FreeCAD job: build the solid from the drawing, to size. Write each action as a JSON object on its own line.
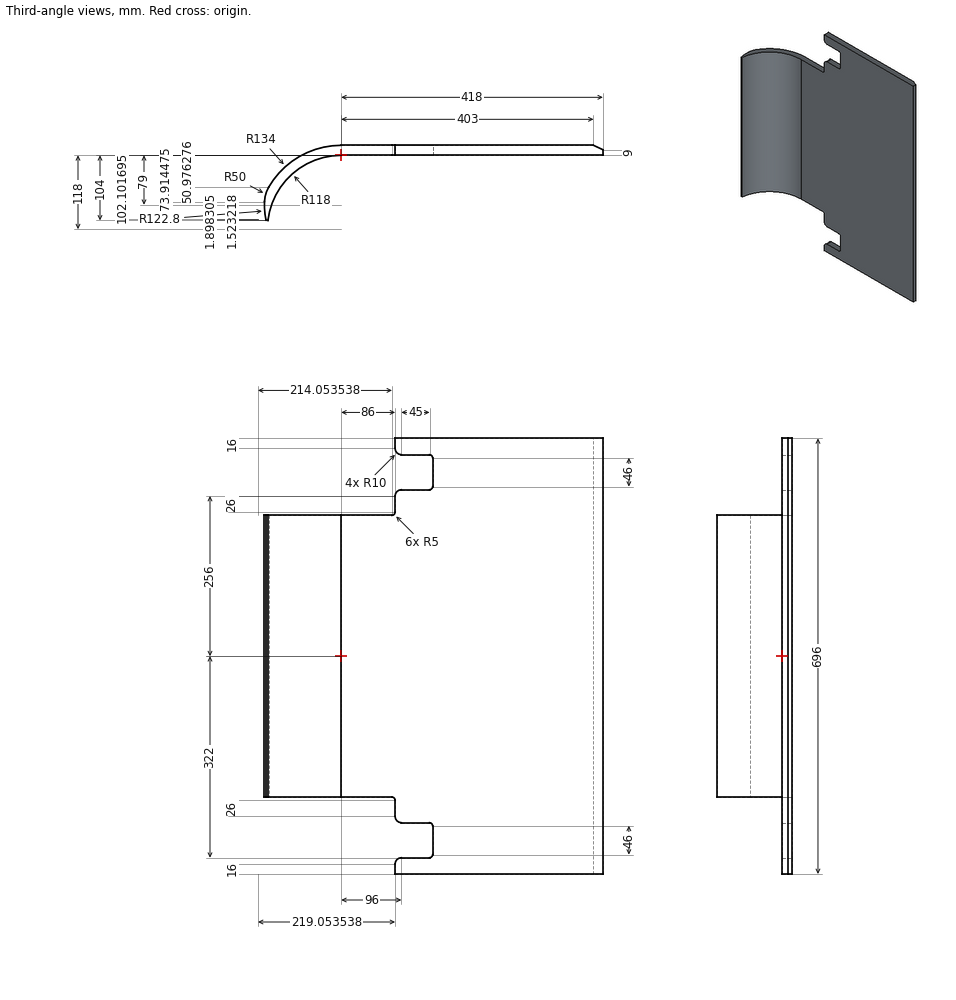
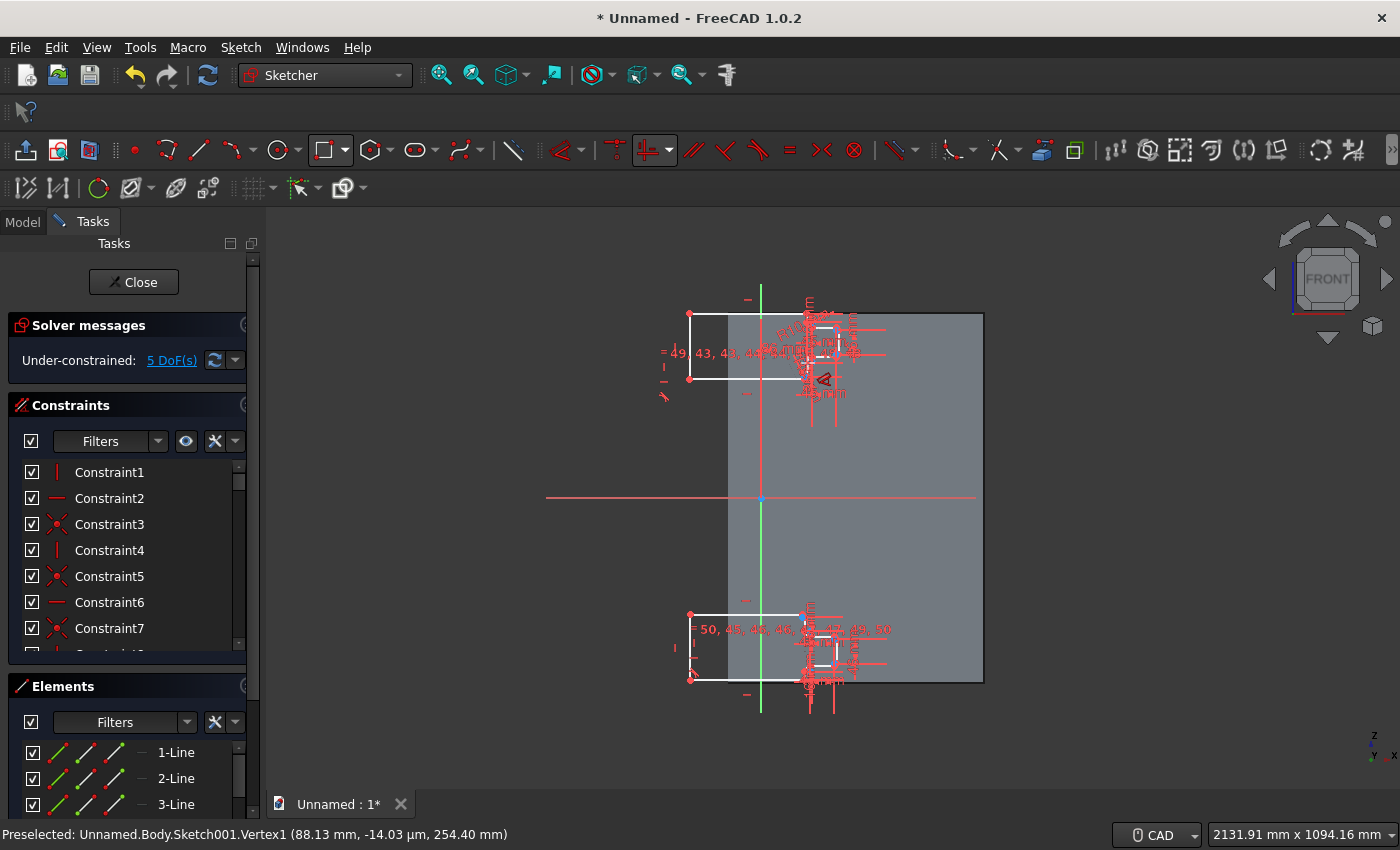
{"action": "scroll", "coordinate": [810, 666], "scroll_direction": "up", "scroll_amount": 5}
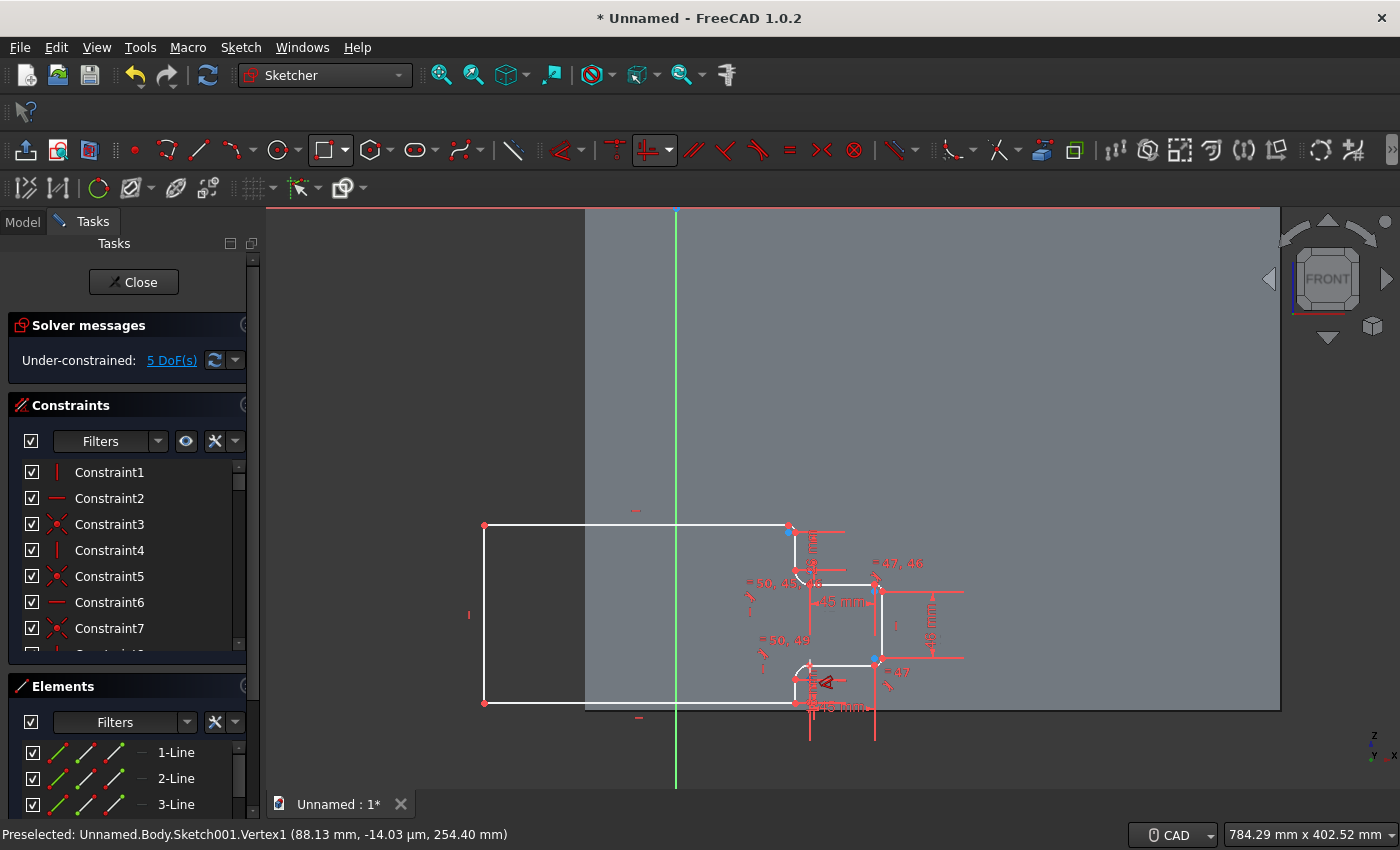
{"action": "left_click", "coordinate": [810, 666]}
{"action": "left_click", "coordinate": [712, 724]}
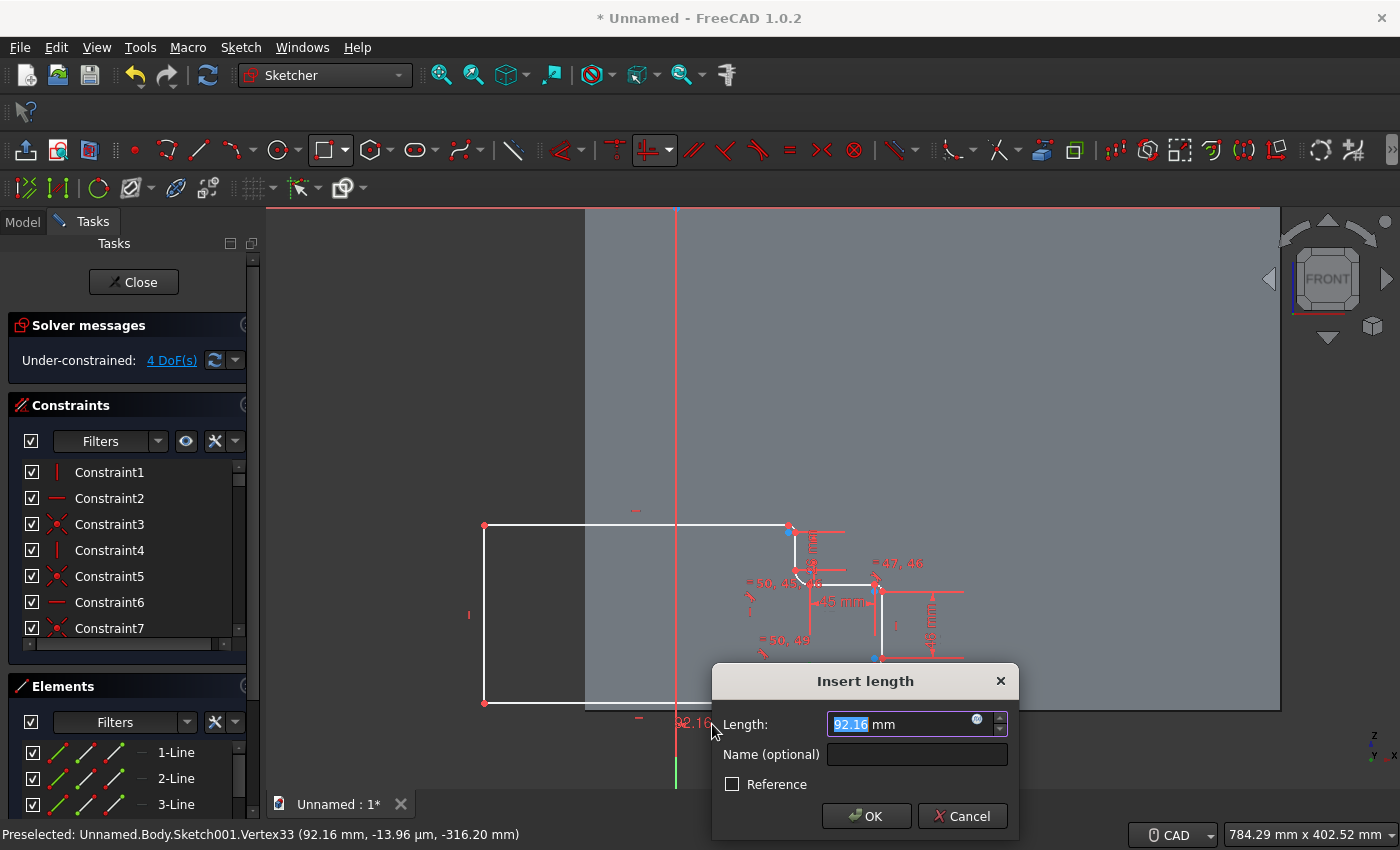
{"action": "type", "text": "96"}
{"action": "key", "text": "Return"}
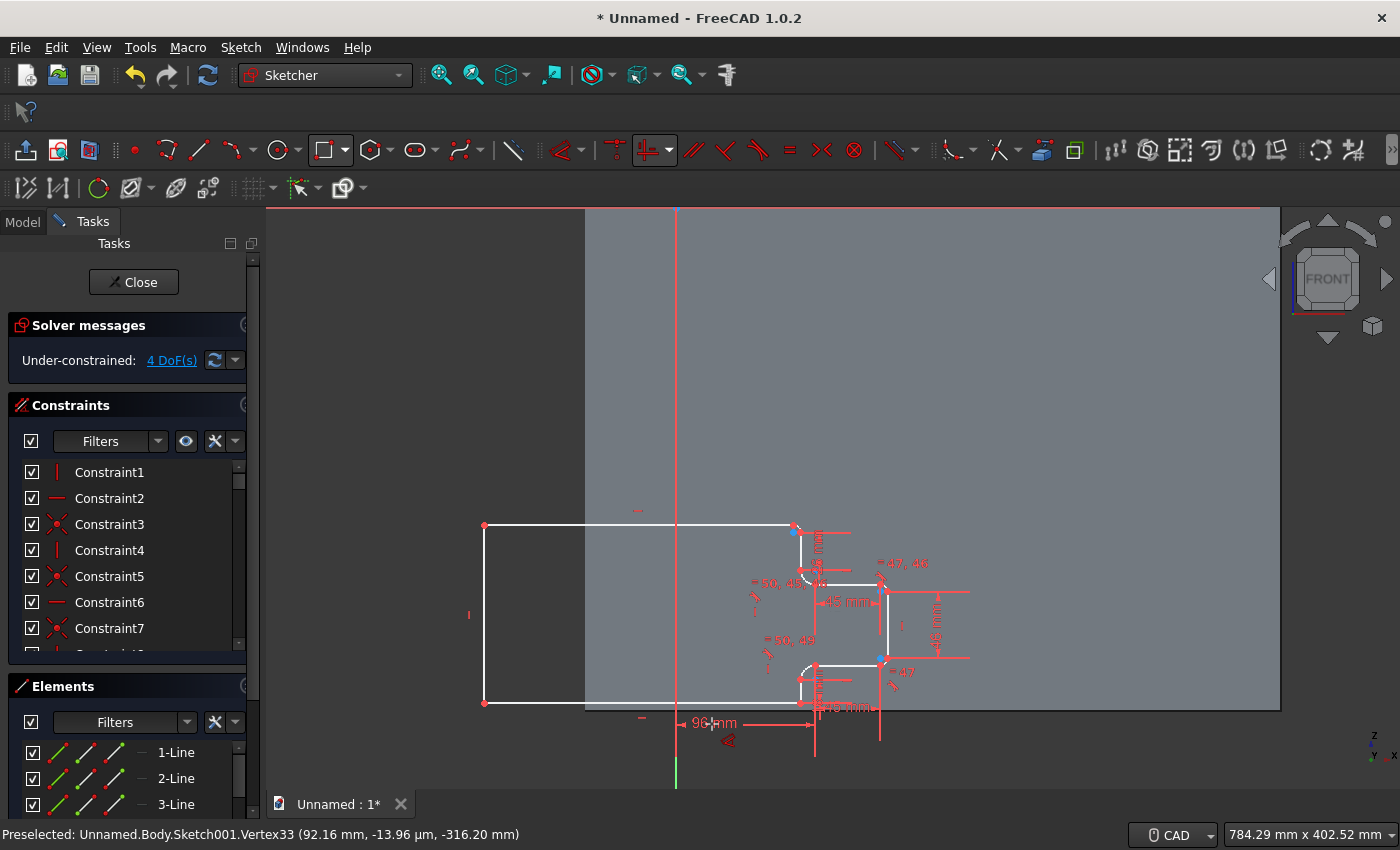
{"action": "scroll", "coordinate": [810, 667], "scroll_direction": "down", "scroll_amount": 5}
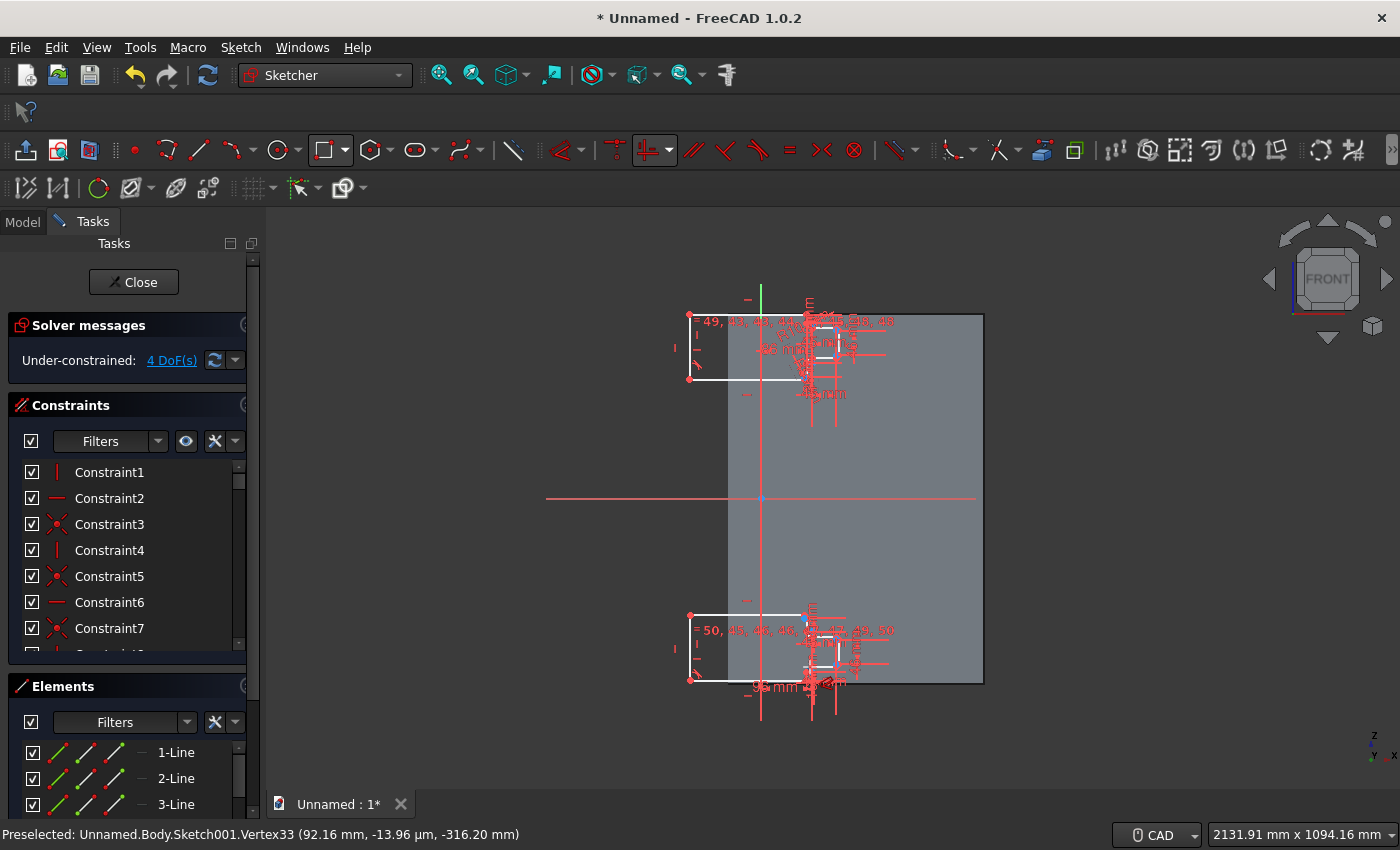
{"action": "scroll", "coordinate": [807, 363], "scroll_direction": "up", "scroll_amount": 5}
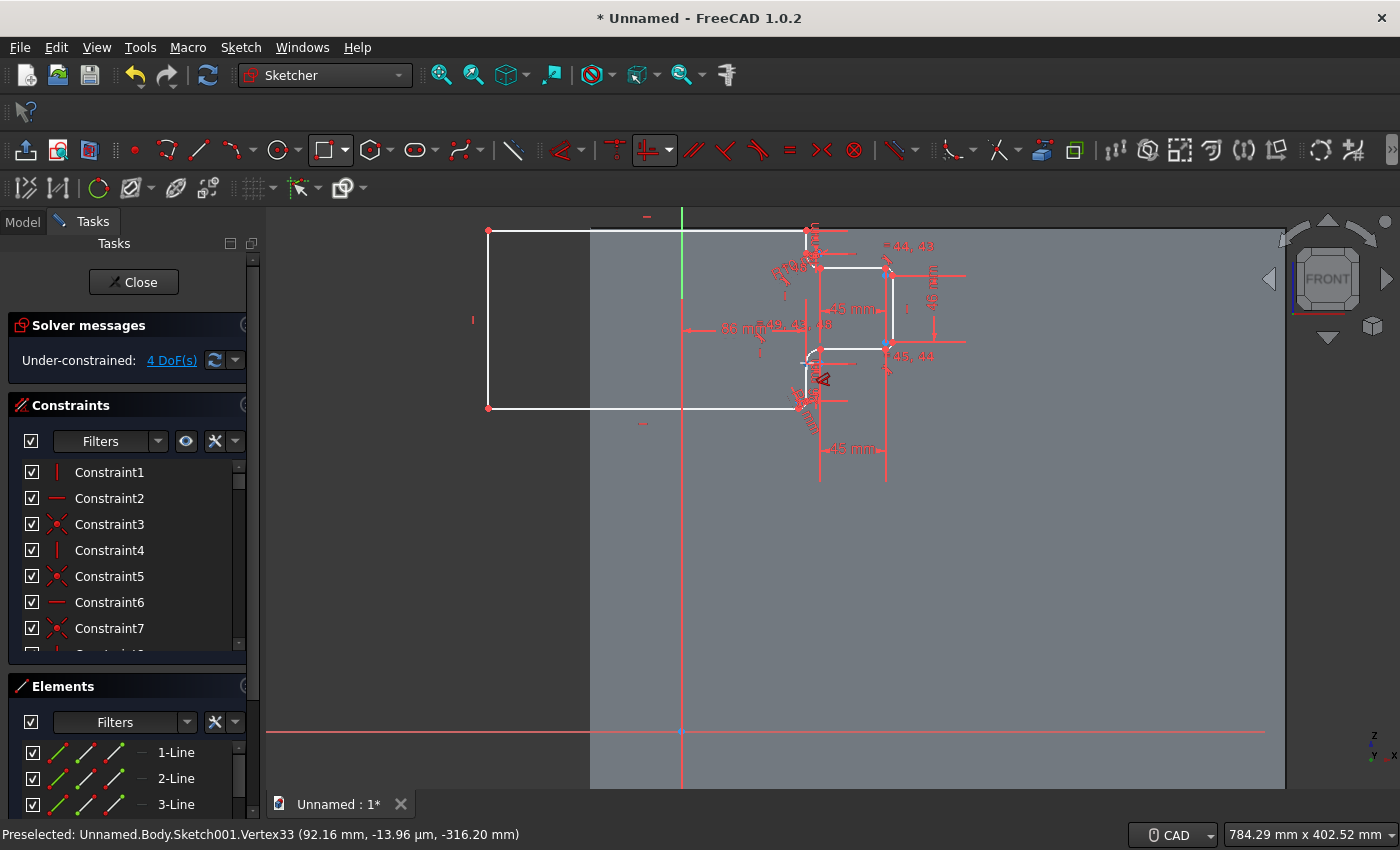
{"action": "left_click", "coordinate": [806, 364]}
{"action": "left_click", "coordinate": [840, 548]}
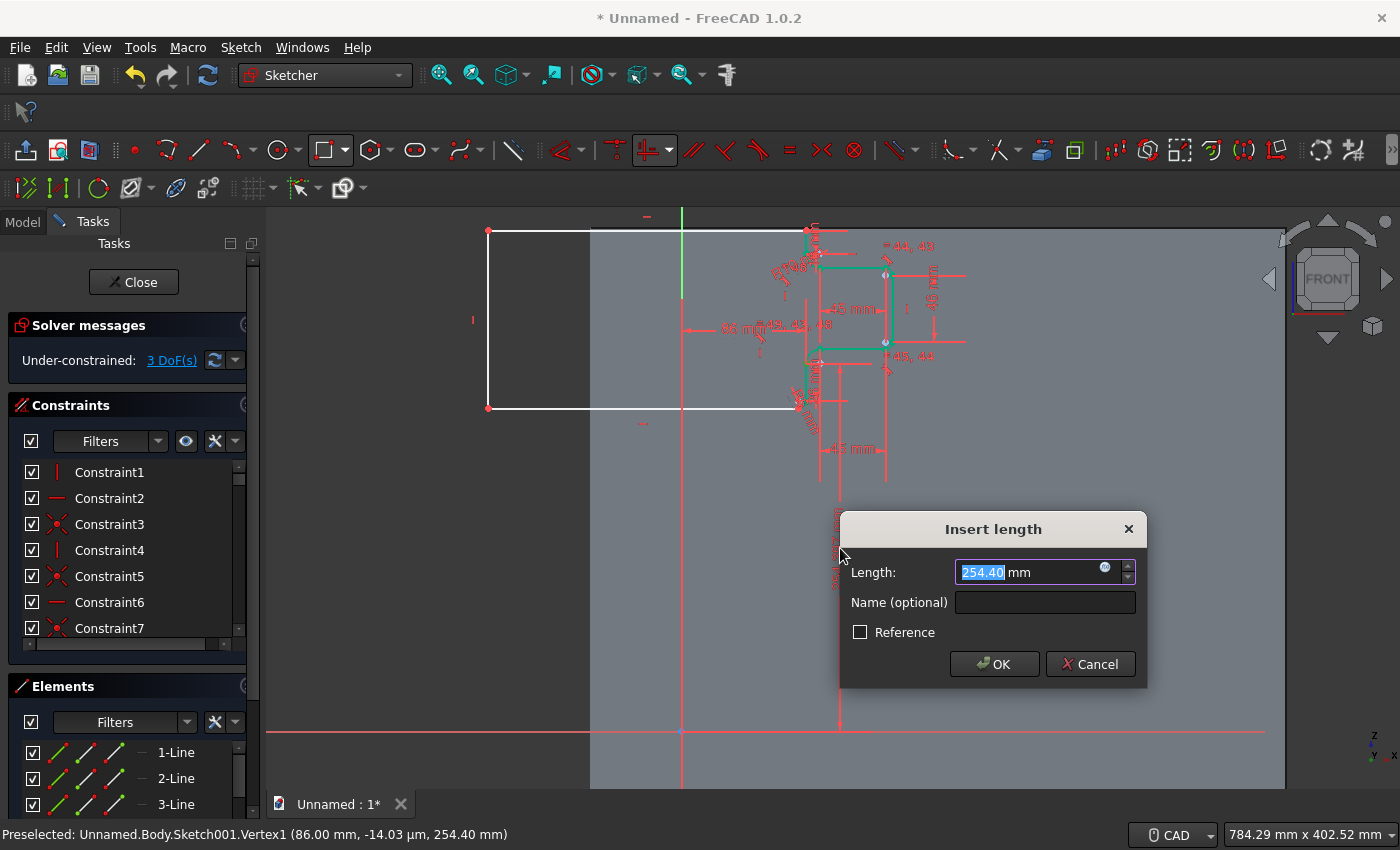
{"action": "type", "text": "256"}
{"action": "key", "text": "Return"}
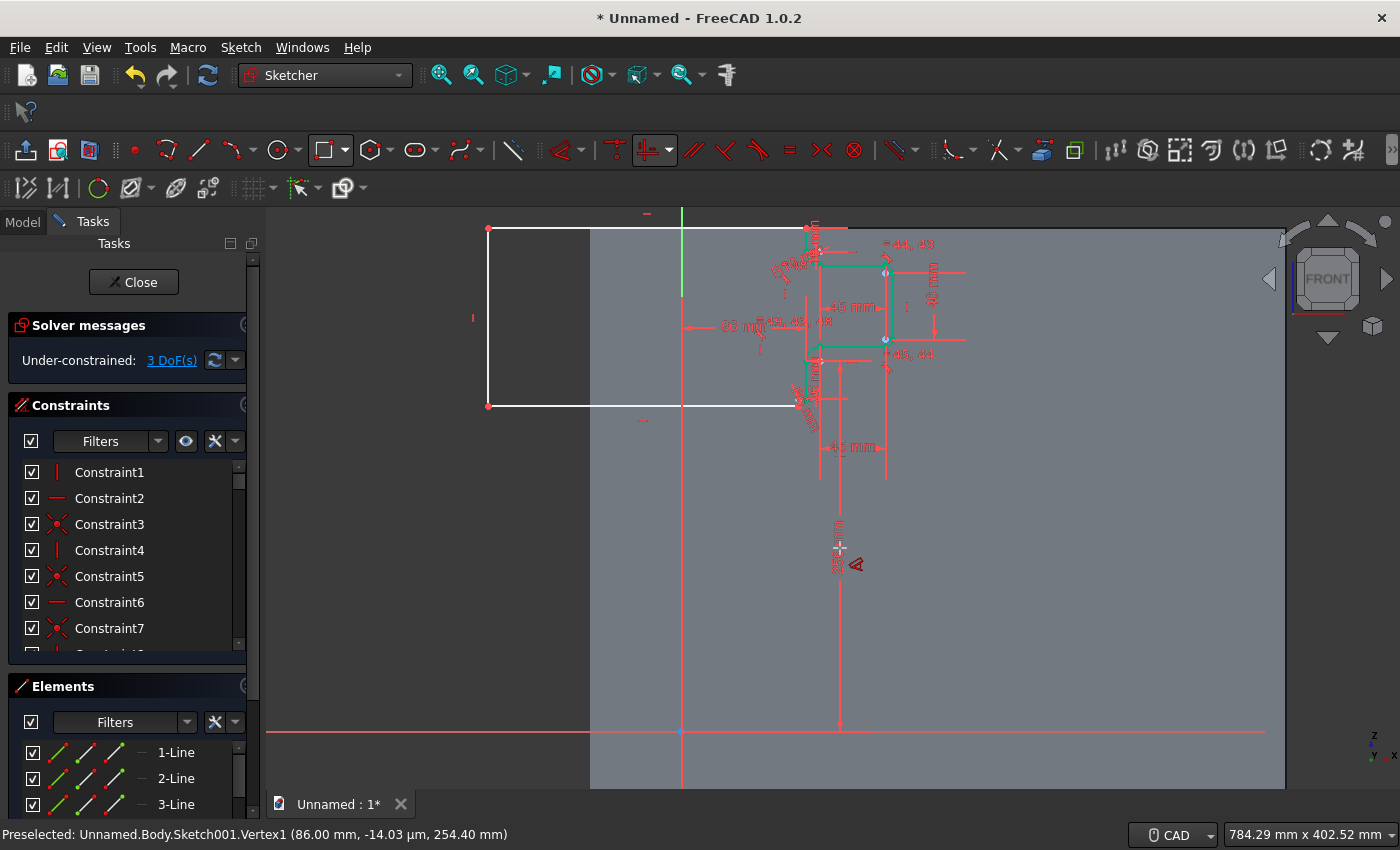
{"action": "scroll", "coordinate": [807, 362], "scroll_direction": "down", "scroll_amount": 5}